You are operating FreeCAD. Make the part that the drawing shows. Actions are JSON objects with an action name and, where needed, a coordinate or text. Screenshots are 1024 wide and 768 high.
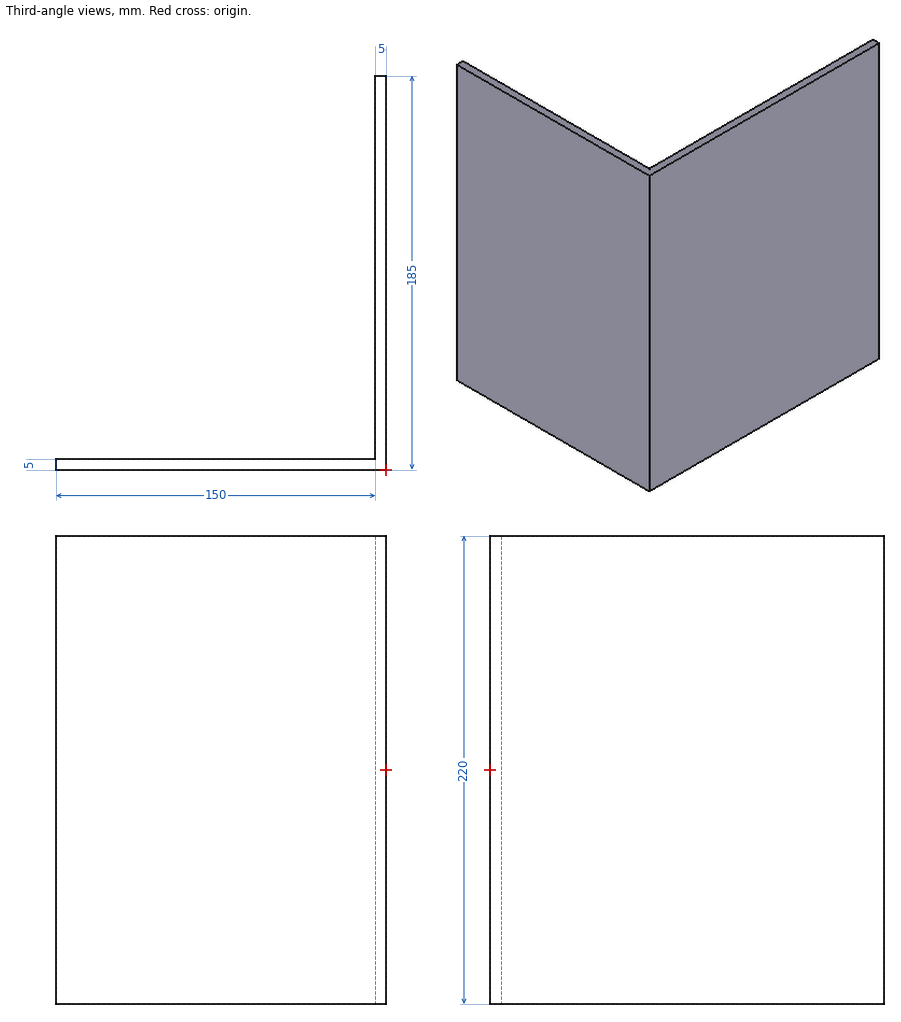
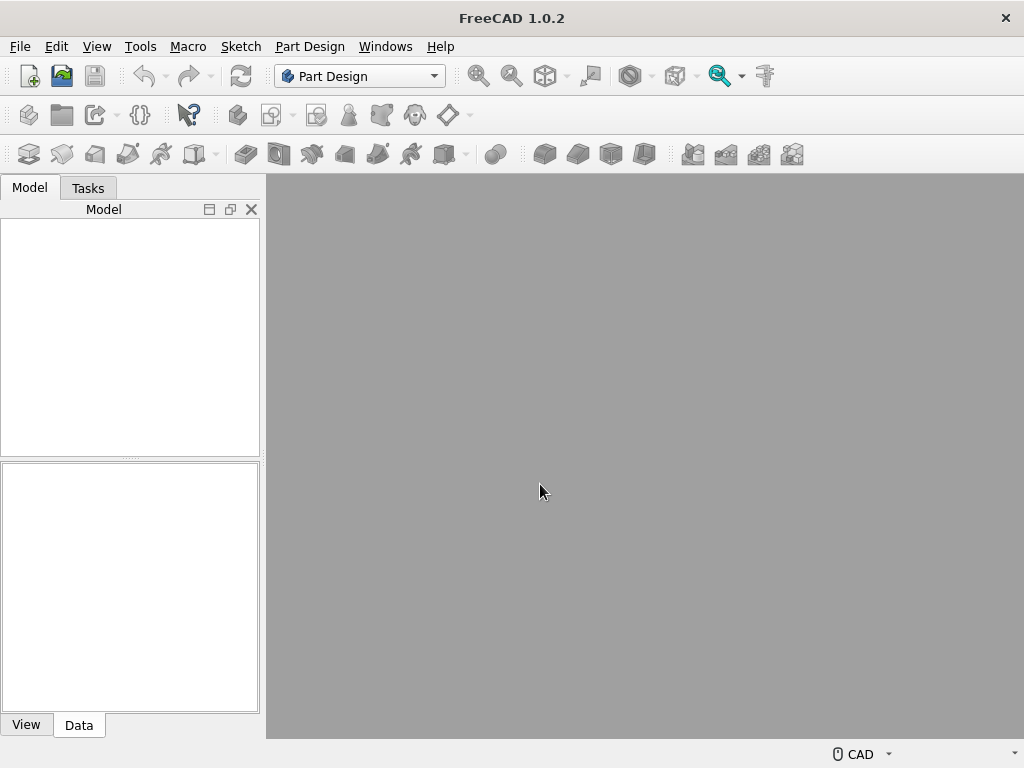
{"action": "left_click", "coordinate": [29, 76]}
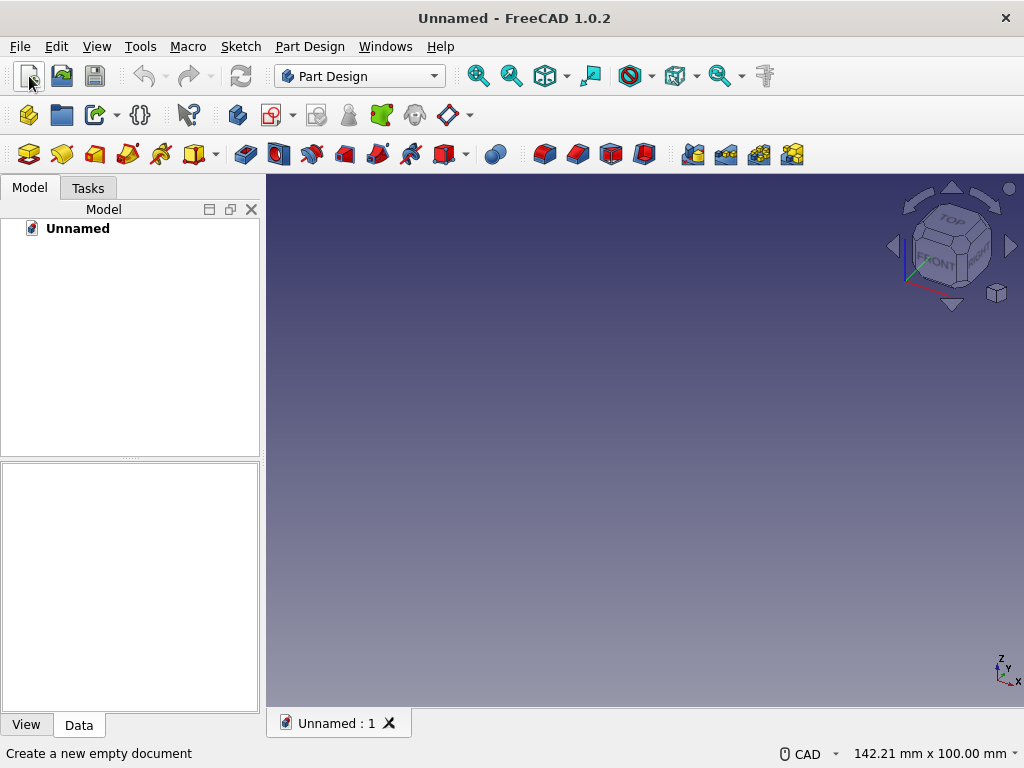
{"action": "left_click", "coordinate": [270, 116]}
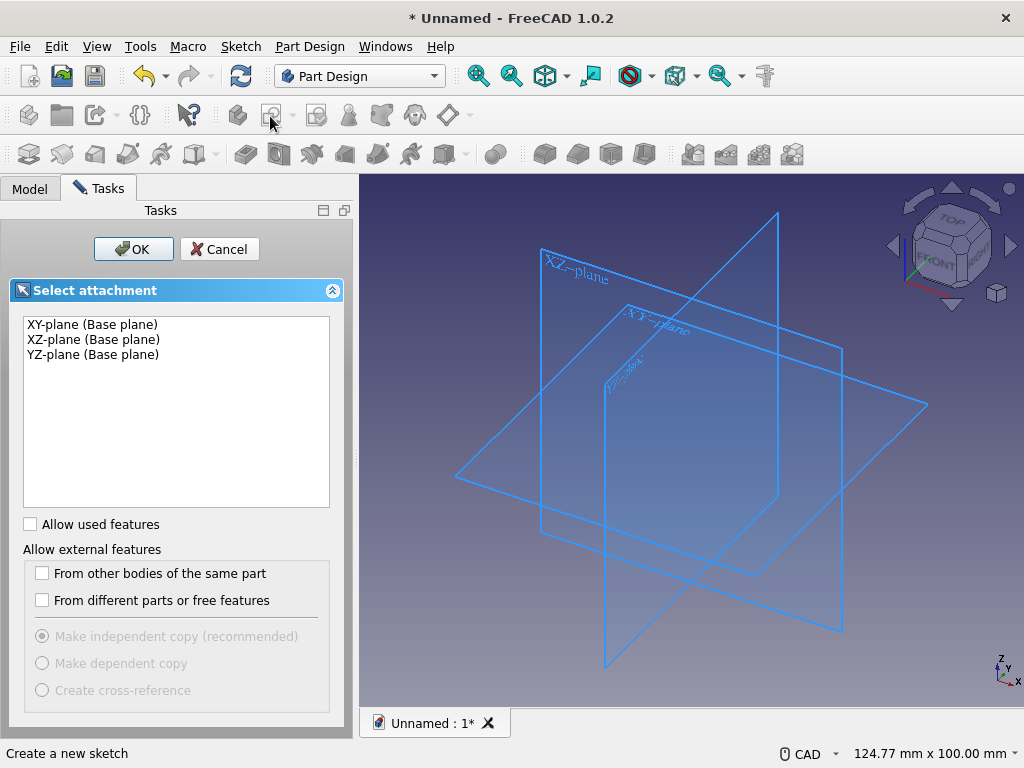
{"action": "left_click", "coordinate": [84, 324]}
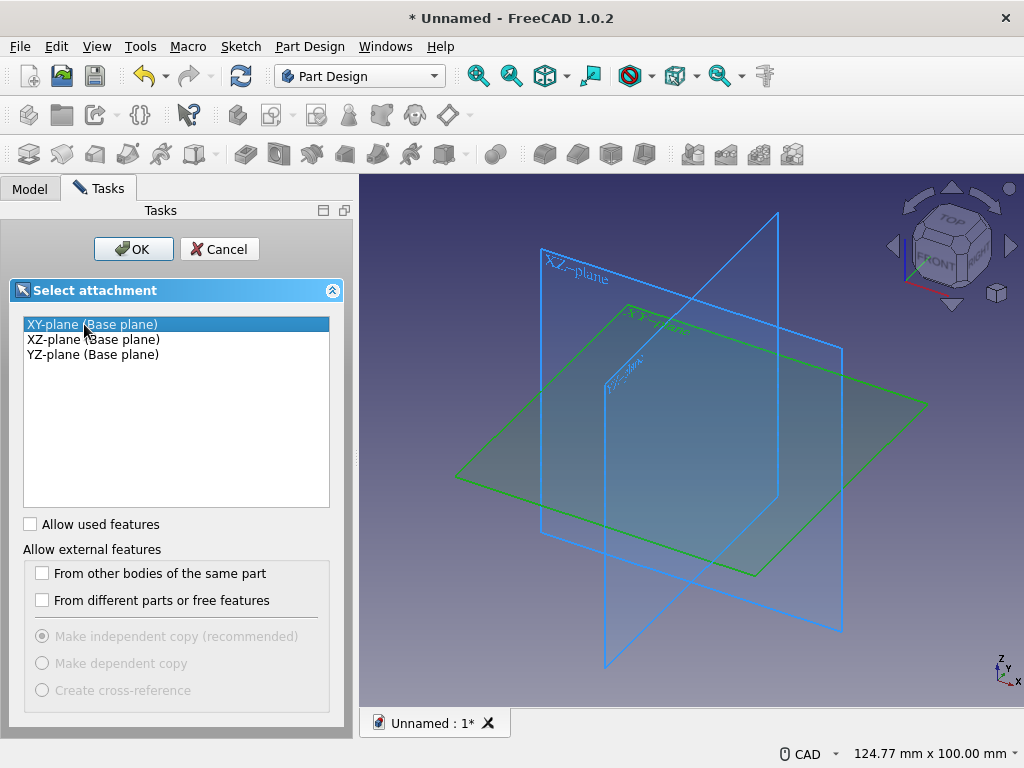
{"action": "left_click", "coordinate": [134, 249]}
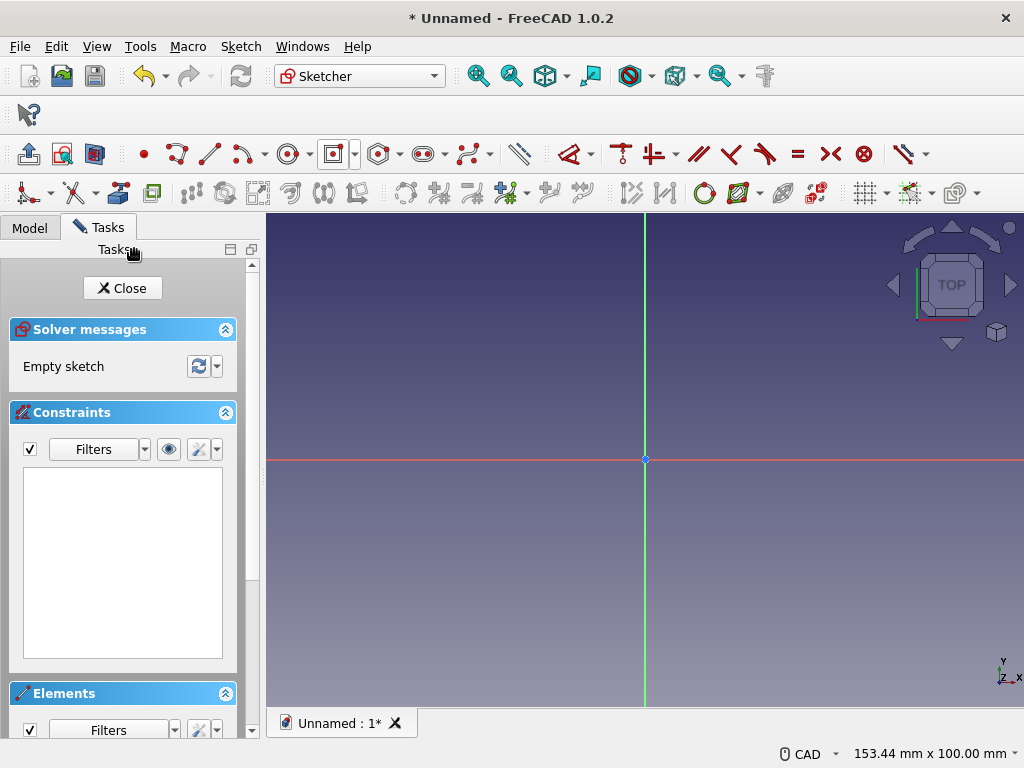
{"action": "scroll", "coordinate": [712, 657], "scroll_direction": "down", "scroll_amount": 6}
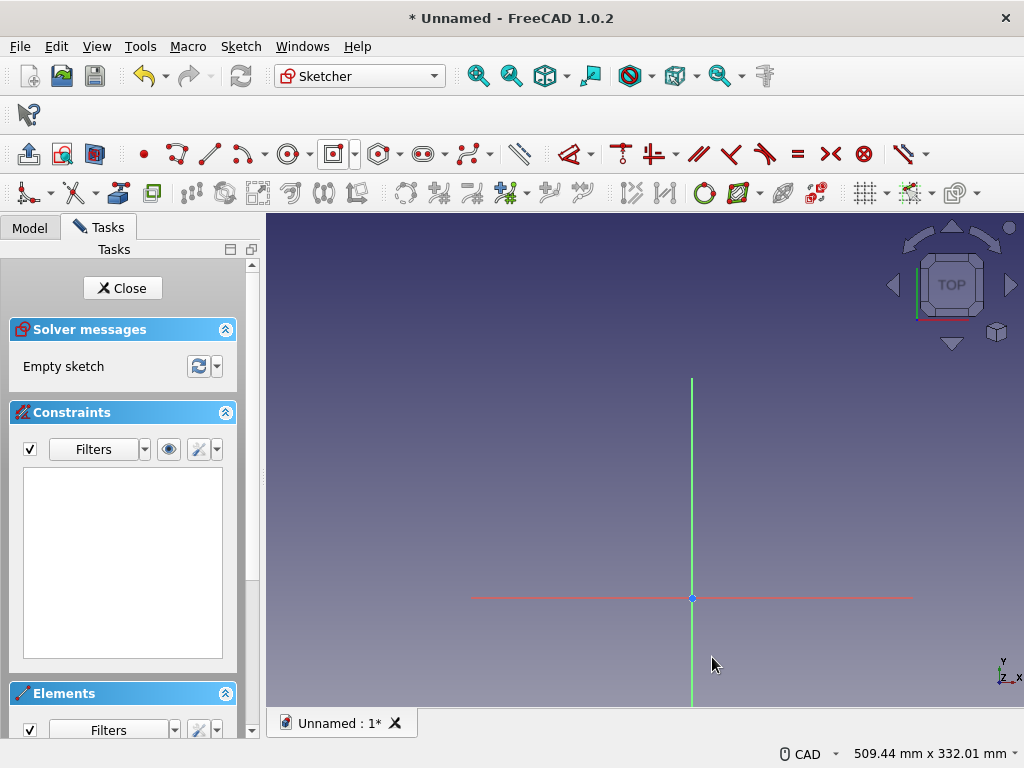
{"action": "left_click", "coordinate": [177, 154]}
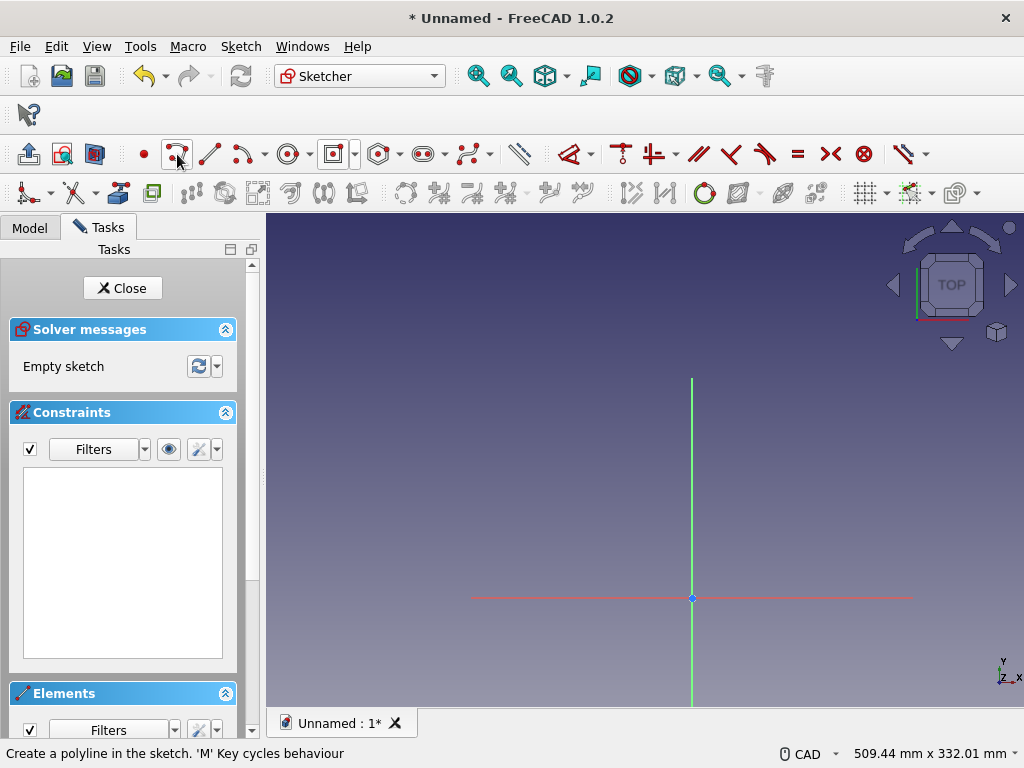
{"action": "left_click", "coordinate": [692, 598]}
{"action": "left_click", "coordinate": [683, 323]}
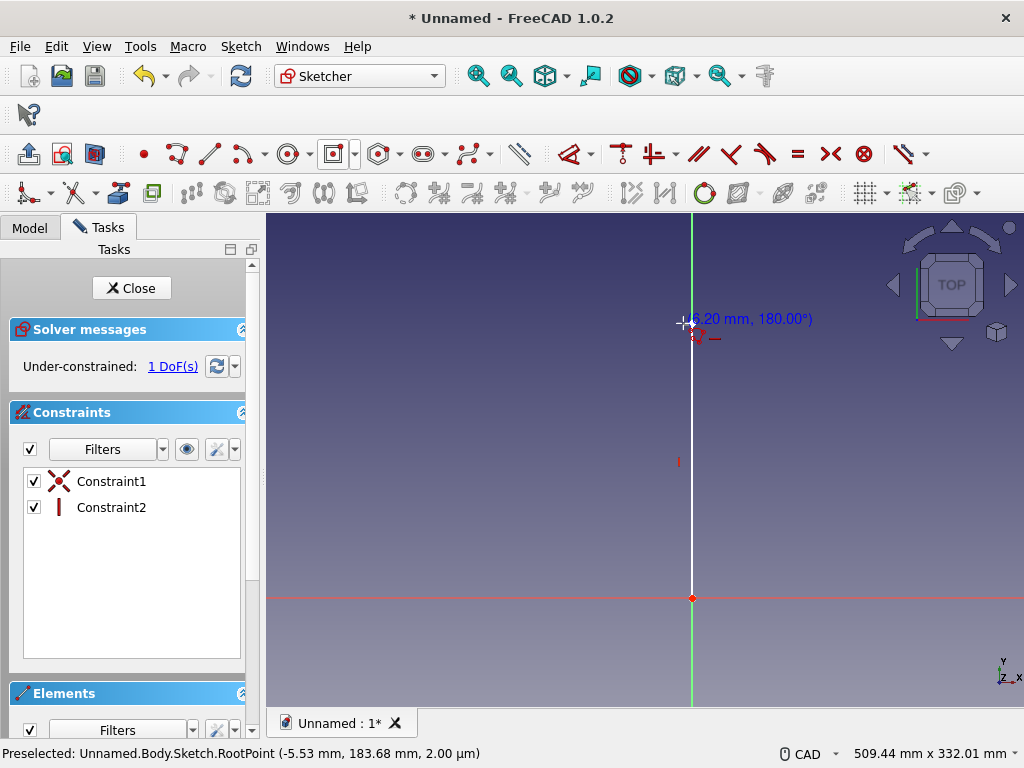
{"action": "scroll", "coordinate": [685, 323], "scroll_direction": "up", "scroll_amount": 4}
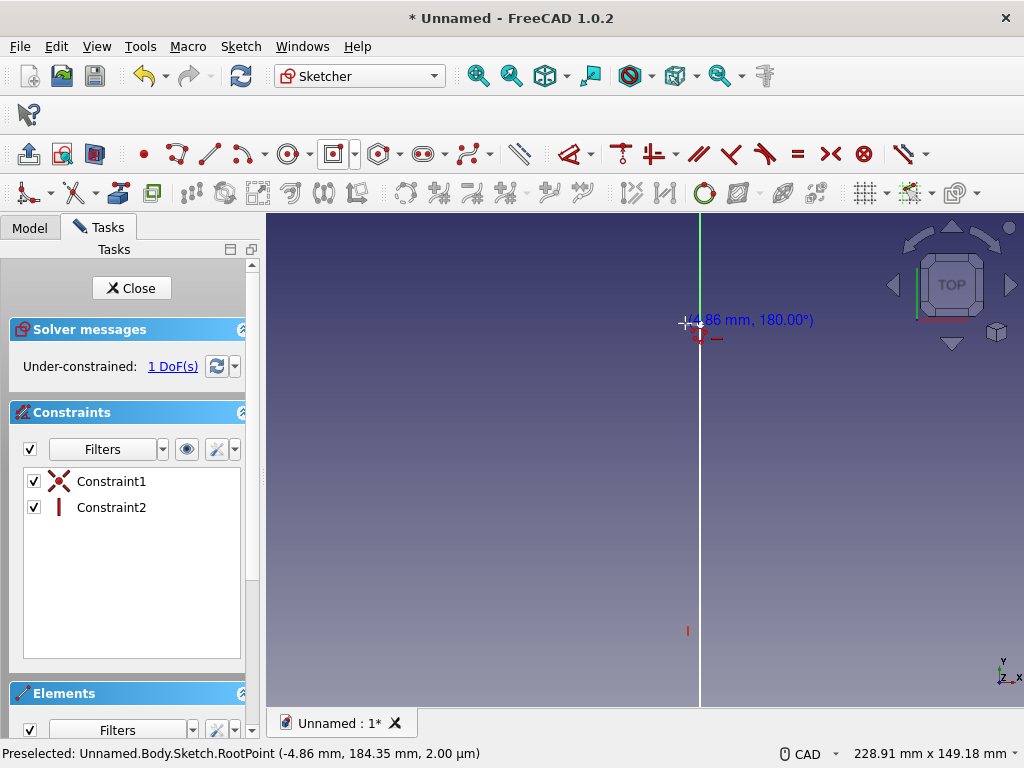
{"action": "left_click", "coordinate": [684, 323]}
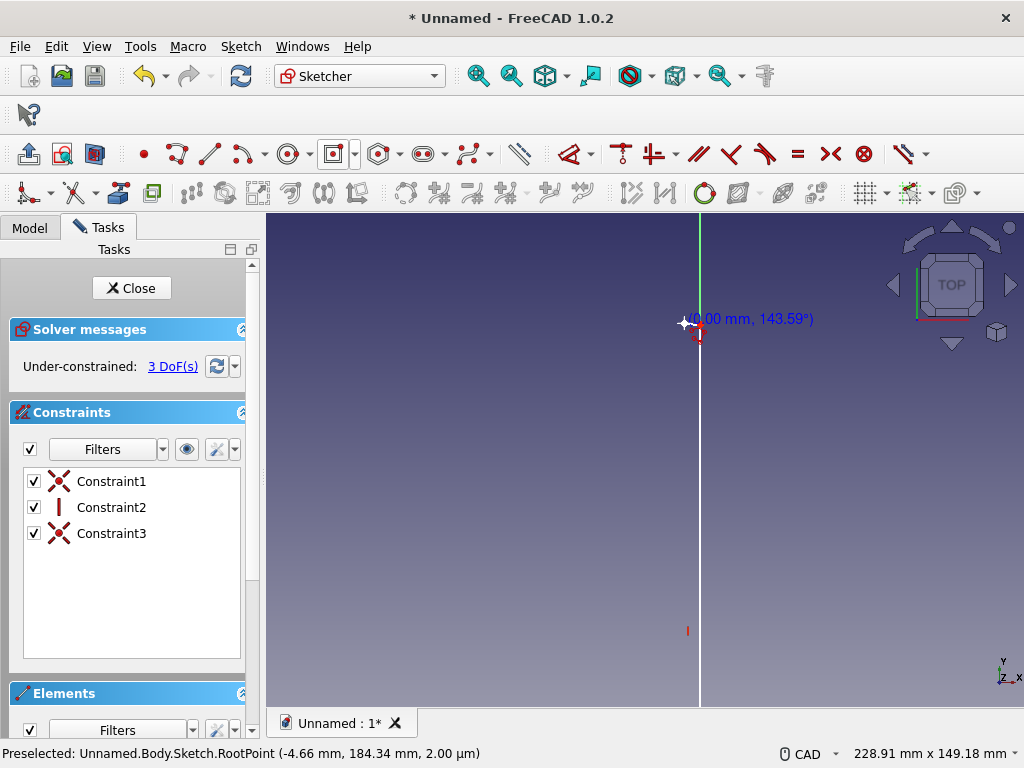
{"action": "scroll", "coordinate": [738, 254], "scroll_direction": "down", "scroll_amount": 3}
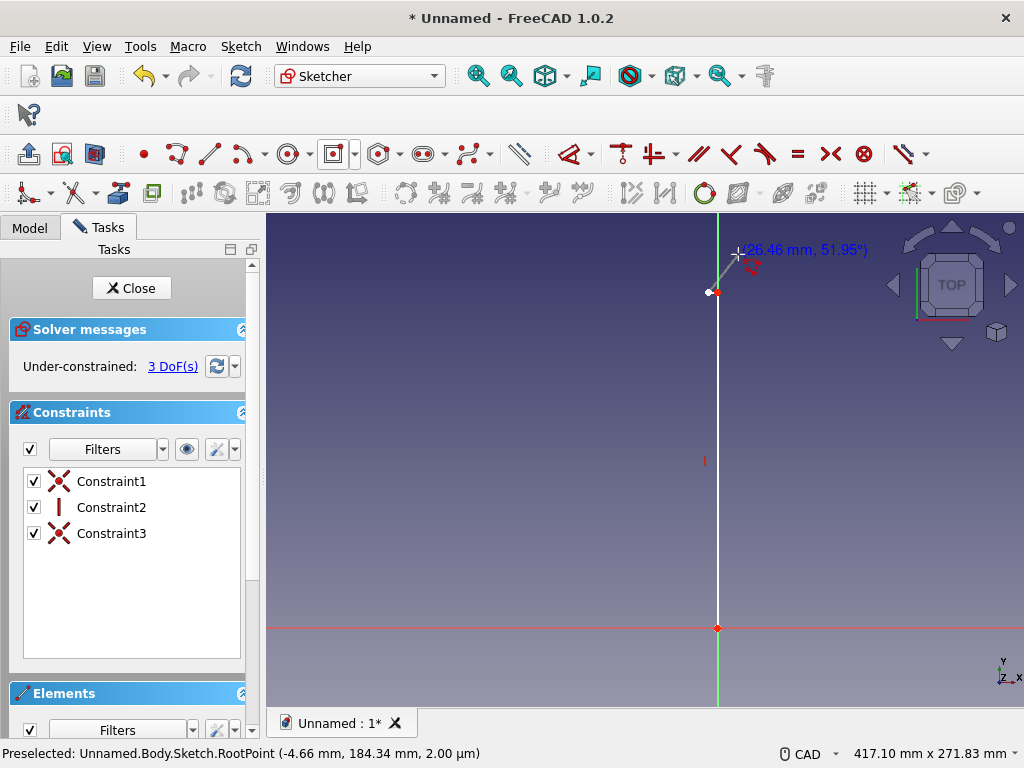
{"action": "scroll", "coordinate": [709, 619], "scroll_direction": "up", "scroll_amount": 3}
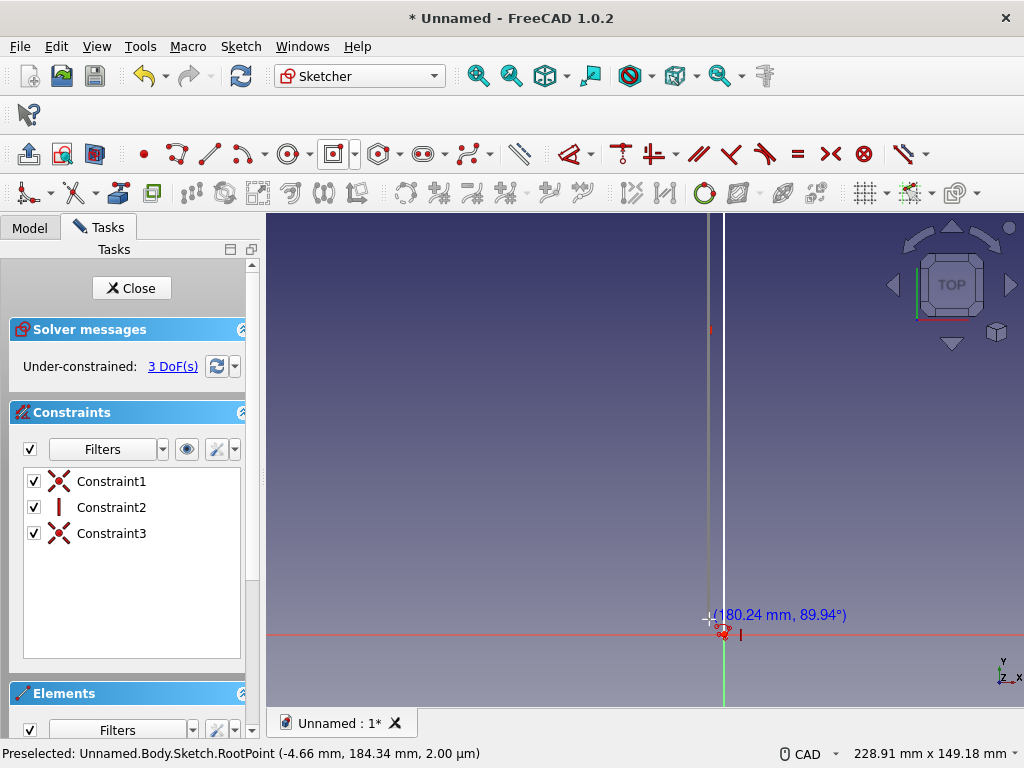
{"action": "left_click", "coordinate": [708, 618]}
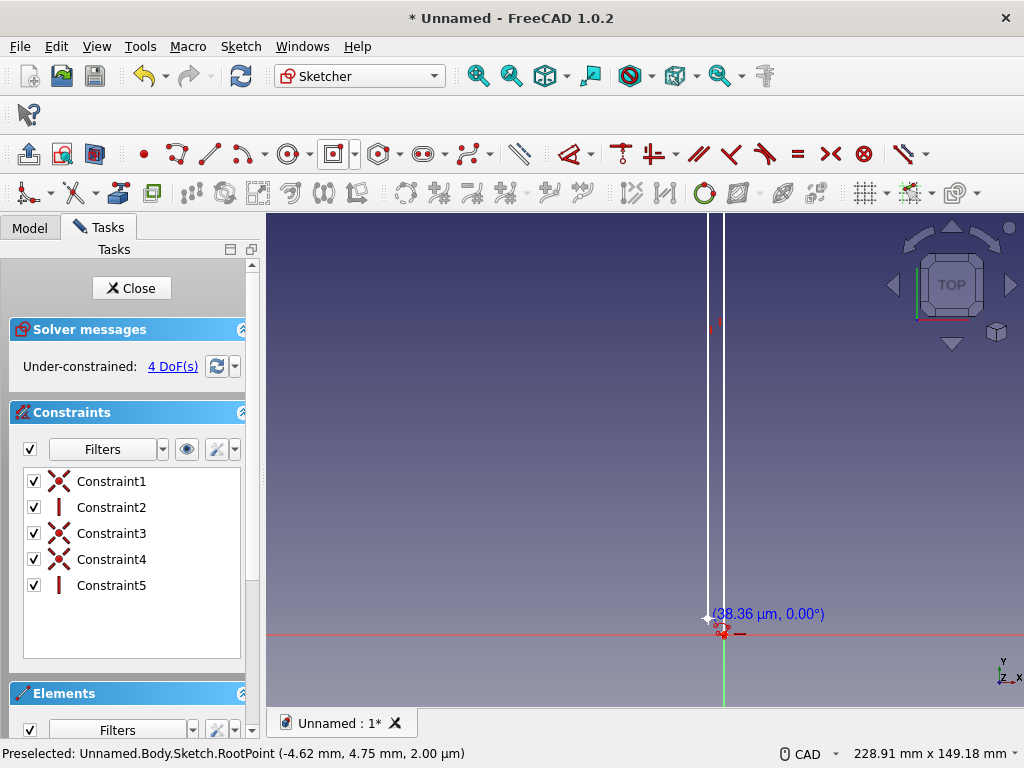
{"action": "scroll", "coordinate": [709, 620], "scroll_direction": "down", "scroll_amount": 3}